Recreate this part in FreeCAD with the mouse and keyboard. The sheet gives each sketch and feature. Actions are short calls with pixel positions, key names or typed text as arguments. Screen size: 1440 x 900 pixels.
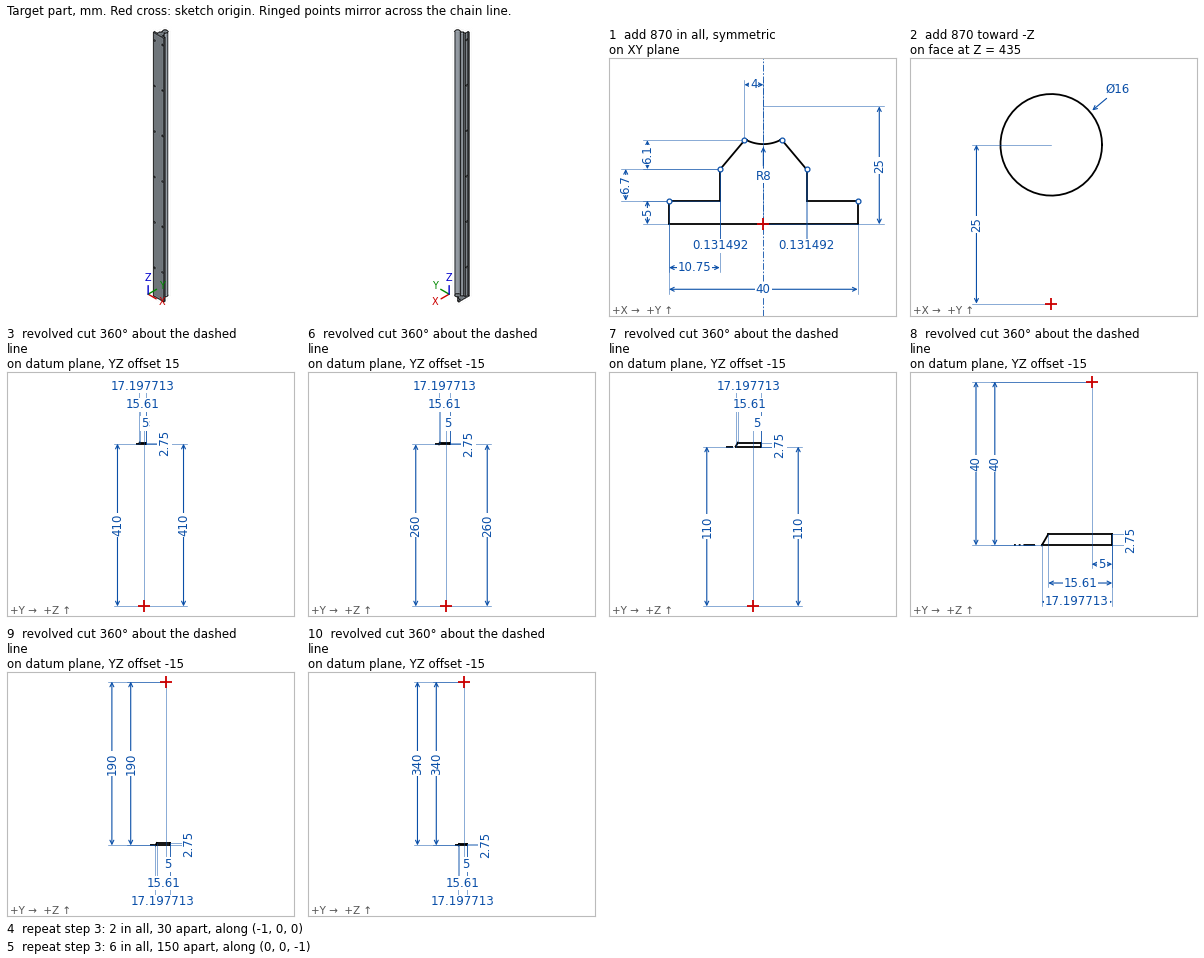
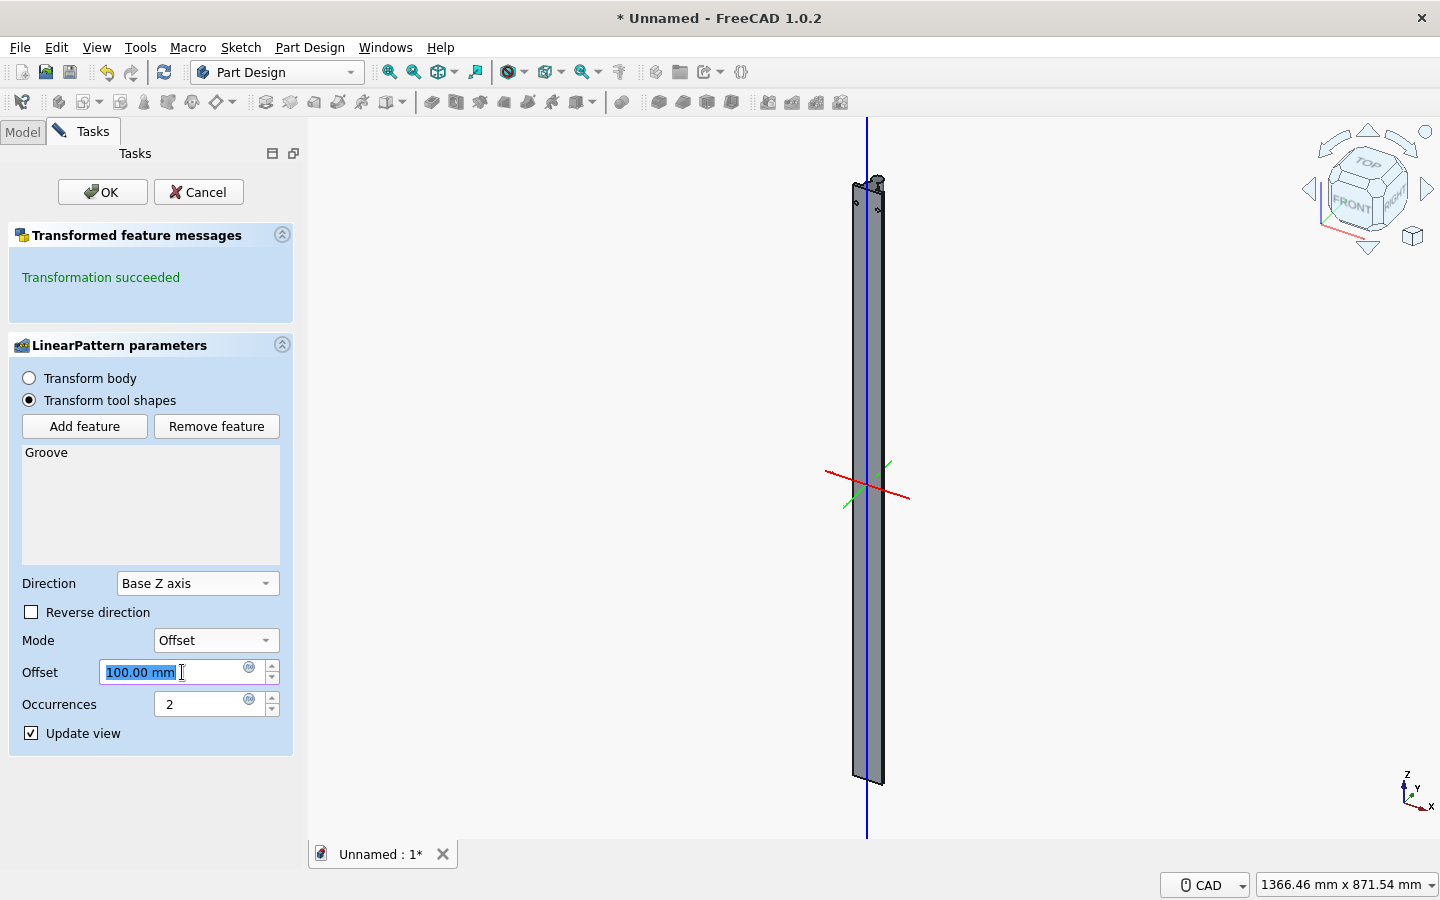
text(150)
key(Tab)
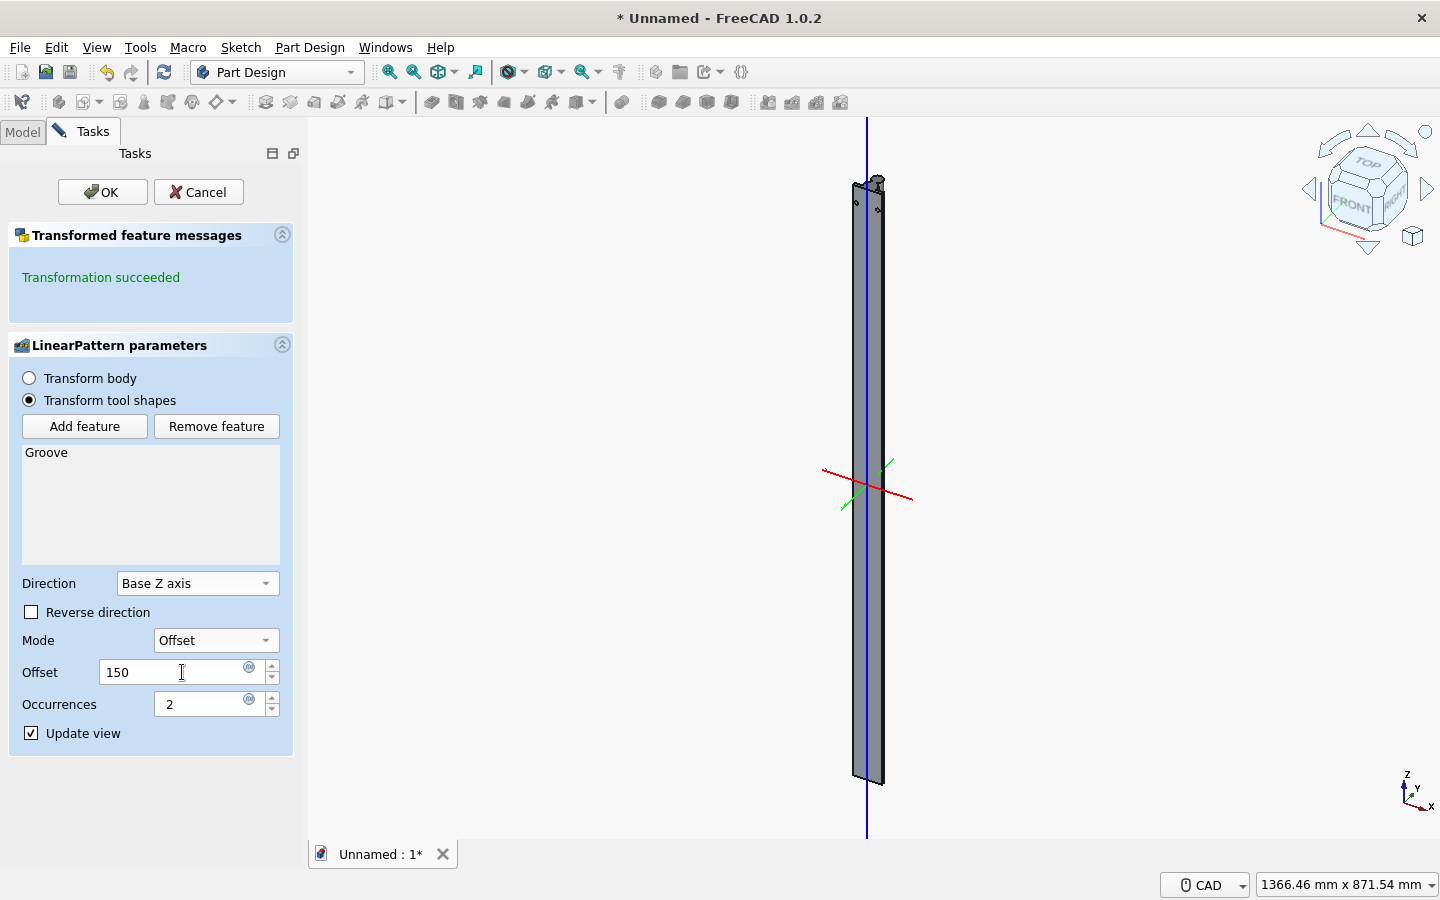
triple_click(209, 704)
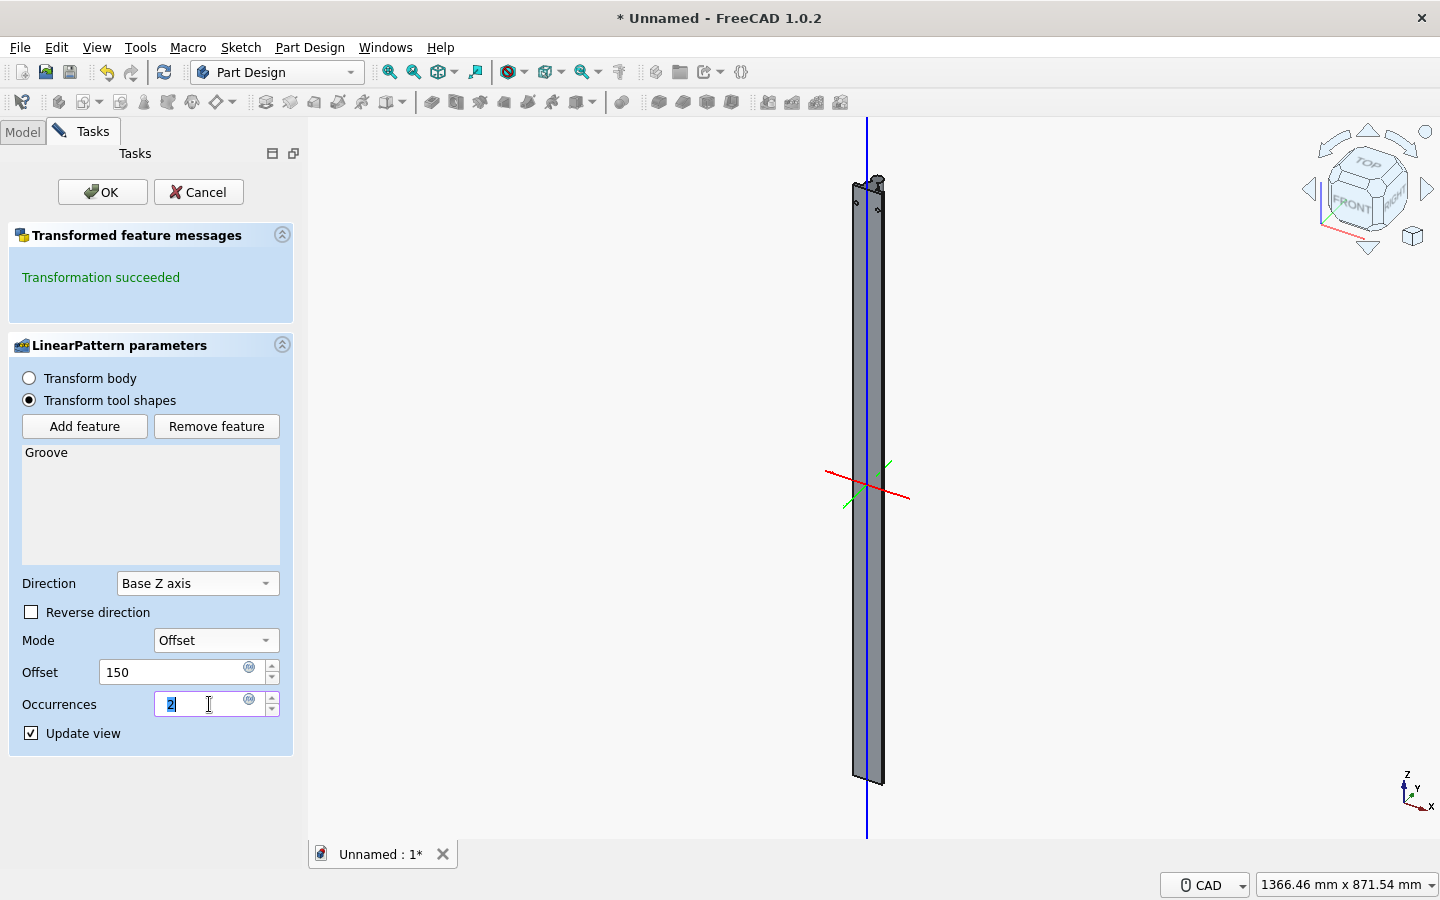
text(6)
key(Tab)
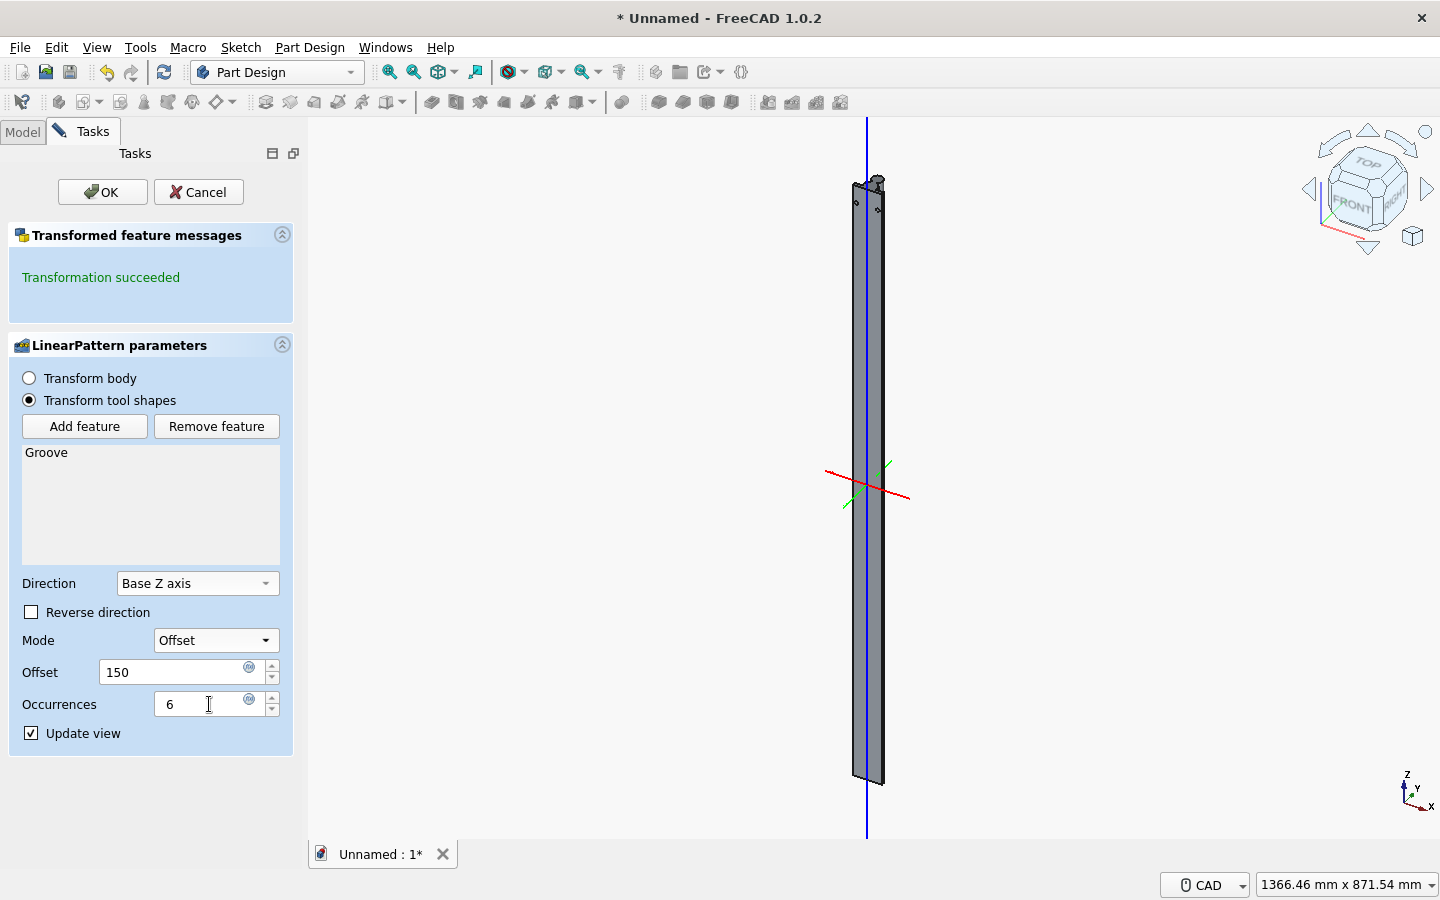
click(30, 612)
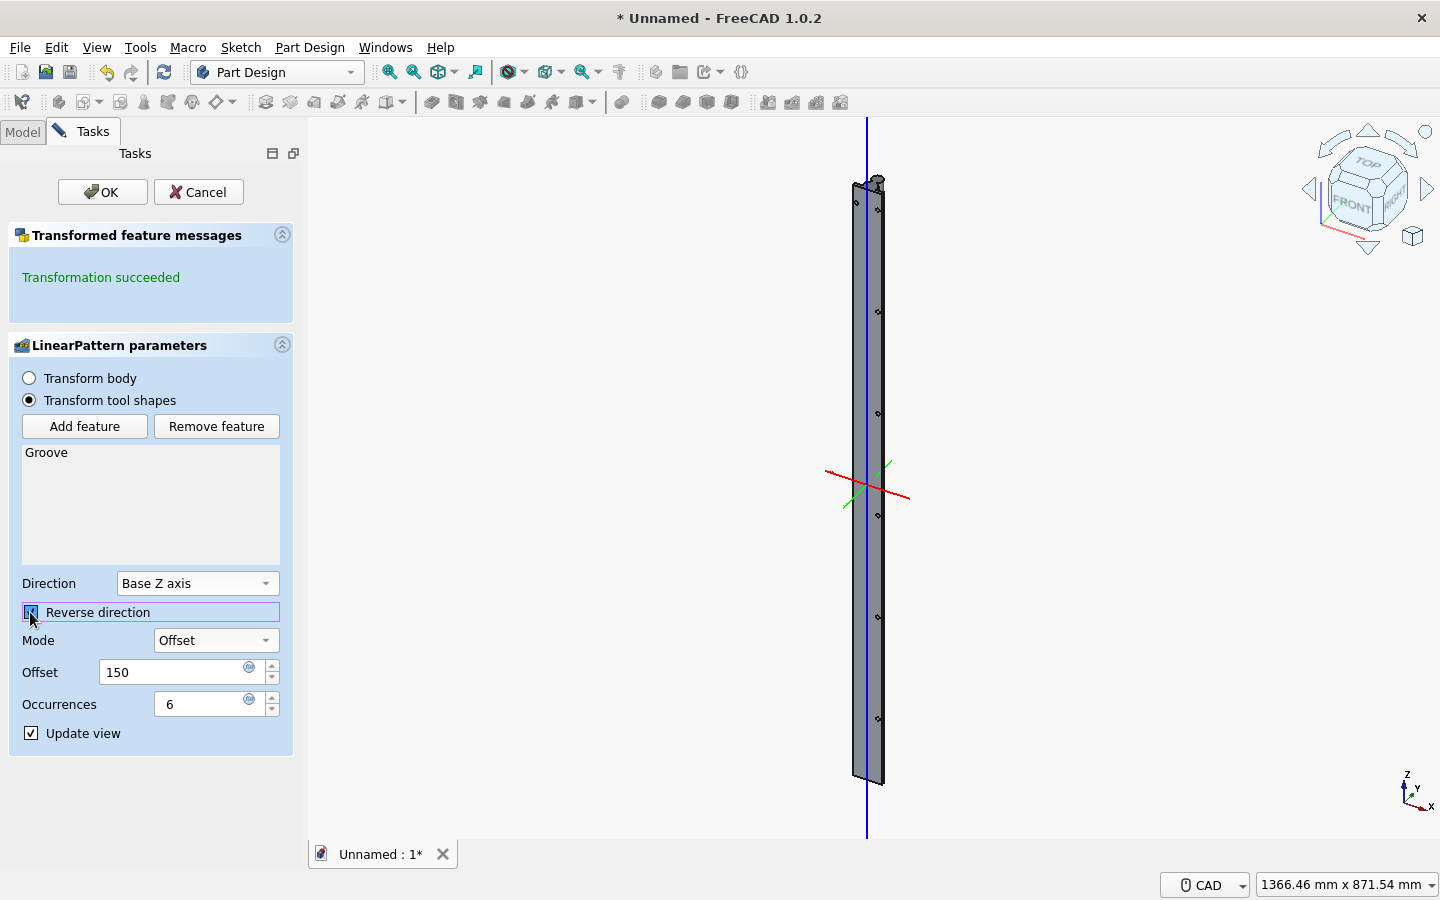
click(103, 192)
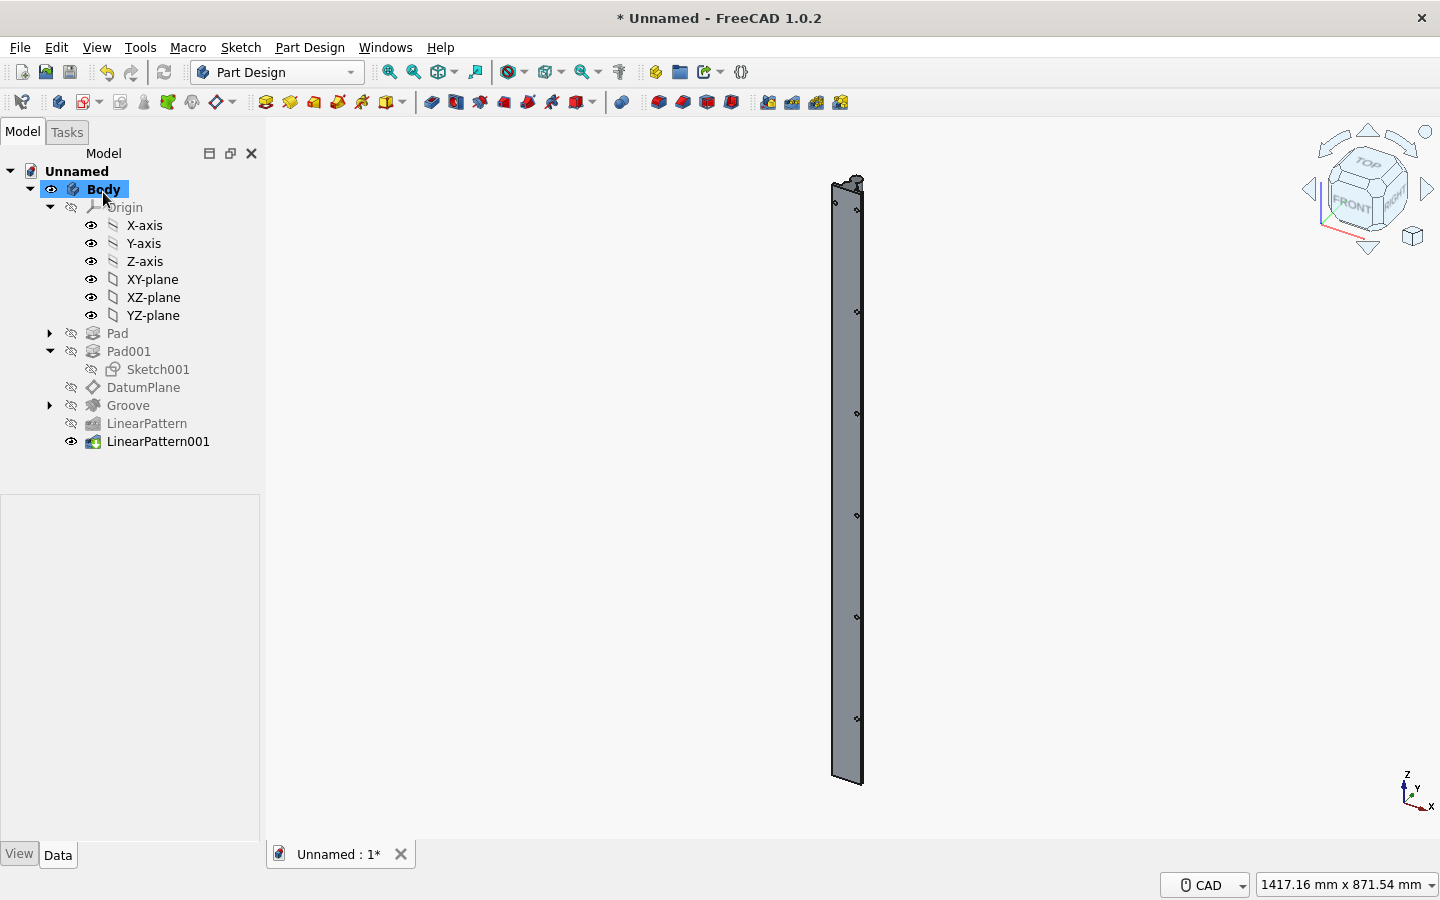
click(136, 315)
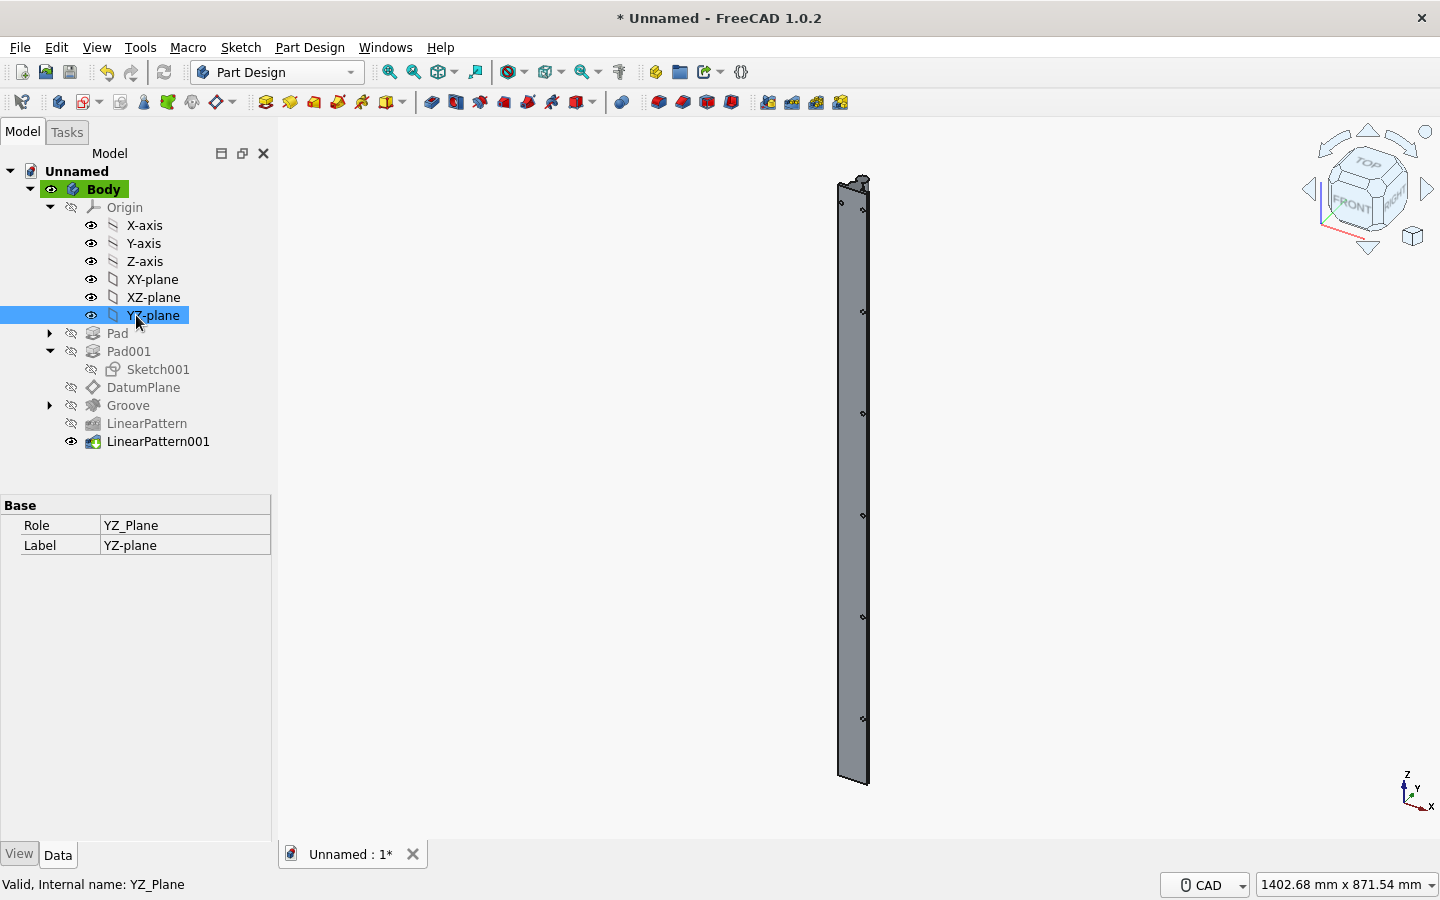
click(216, 102)